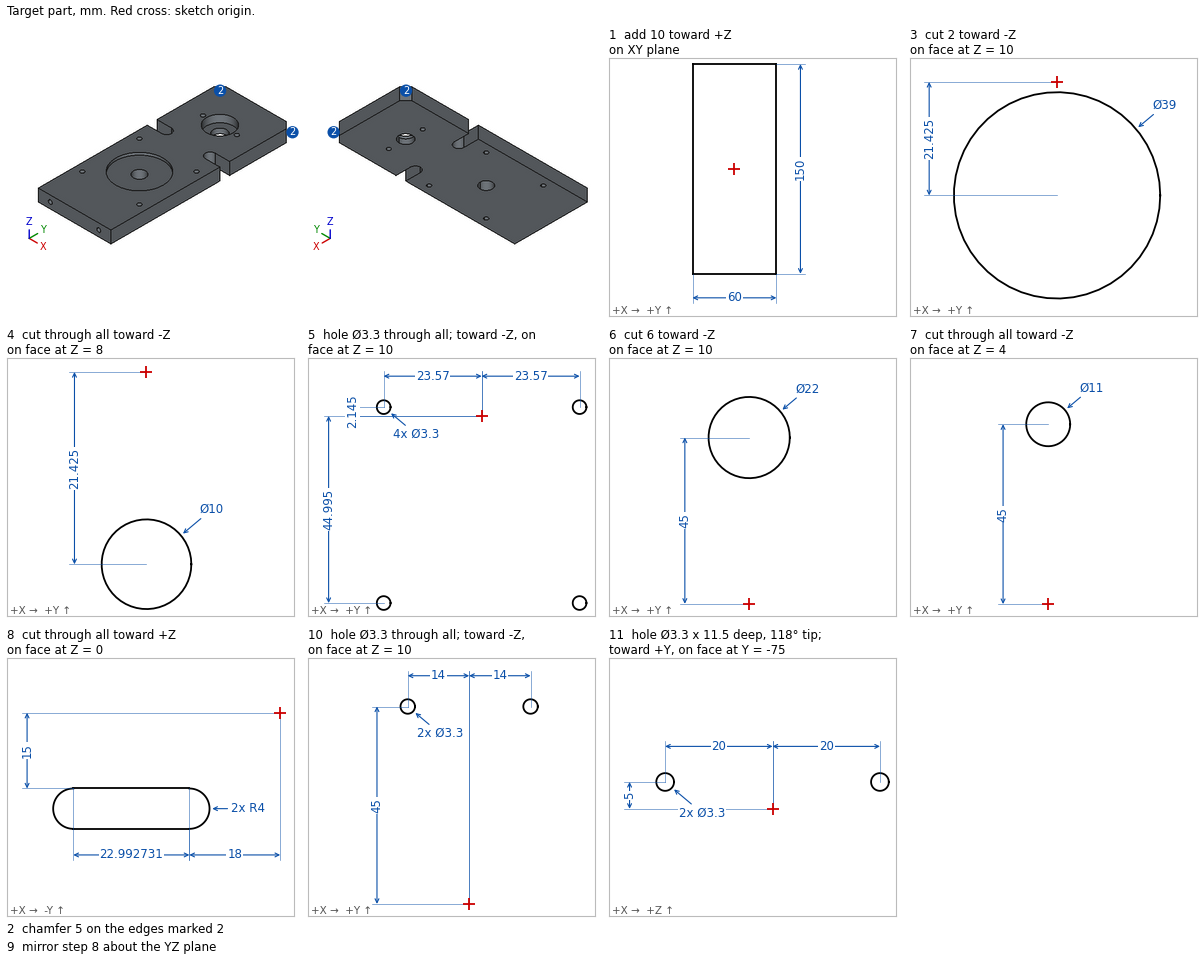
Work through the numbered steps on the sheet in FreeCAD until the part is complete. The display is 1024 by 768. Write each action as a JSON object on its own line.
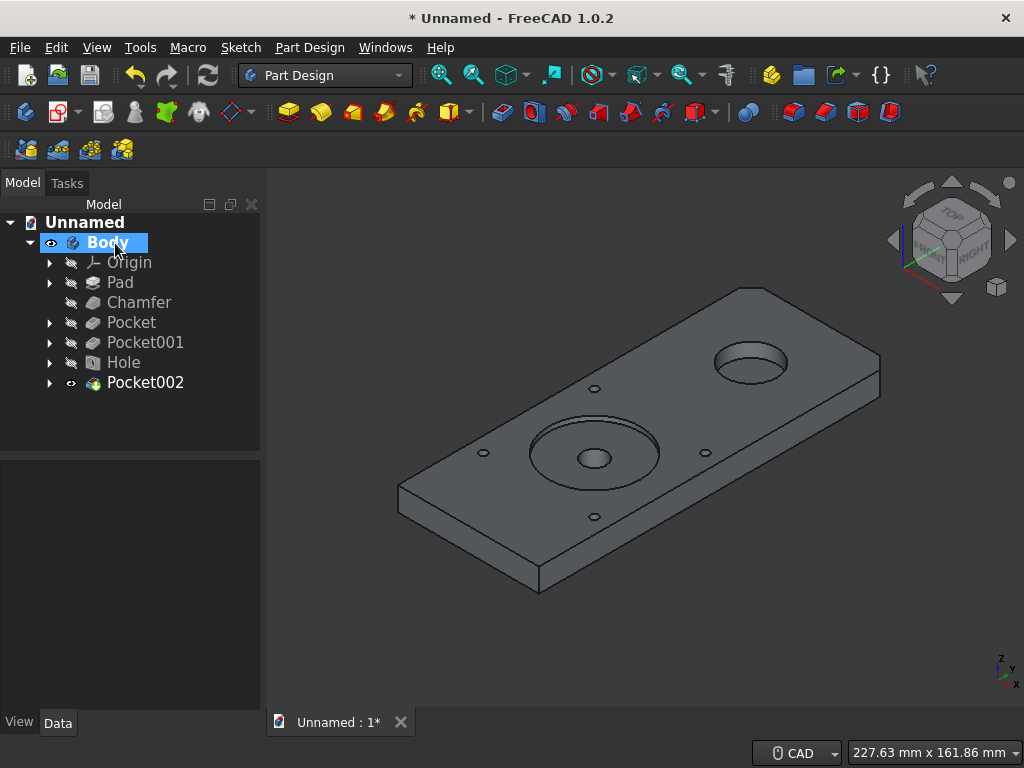
{"action": "left_click", "coordinate": [751, 369]}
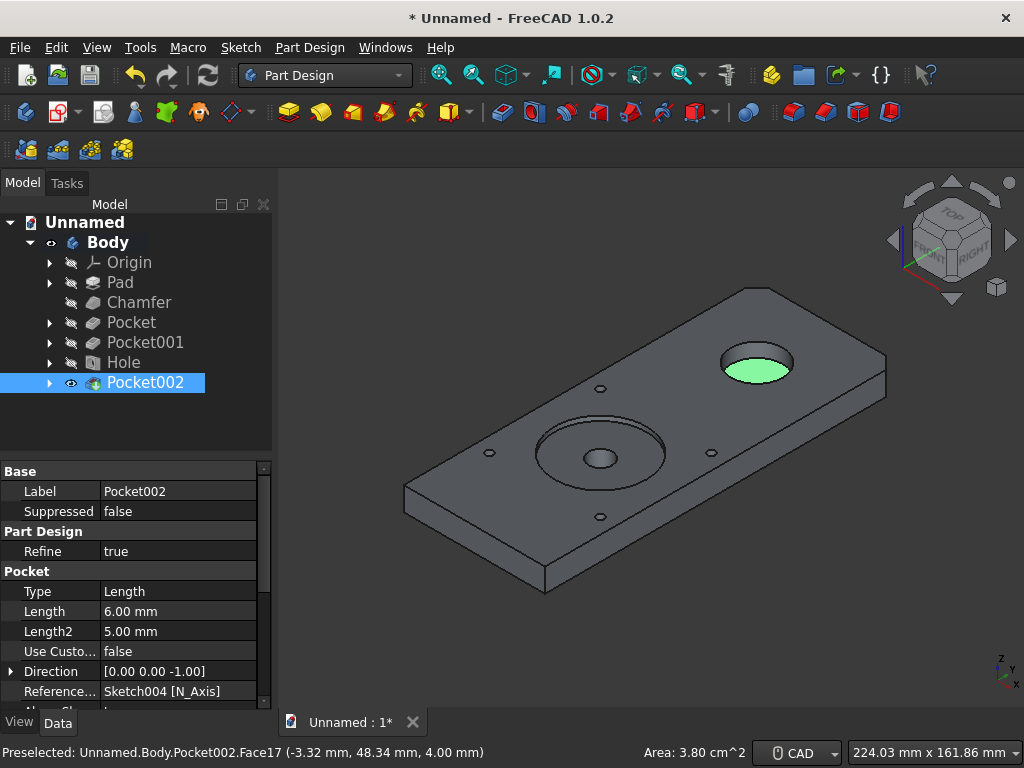
{"action": "left_click", "coordinate": [58, 112]}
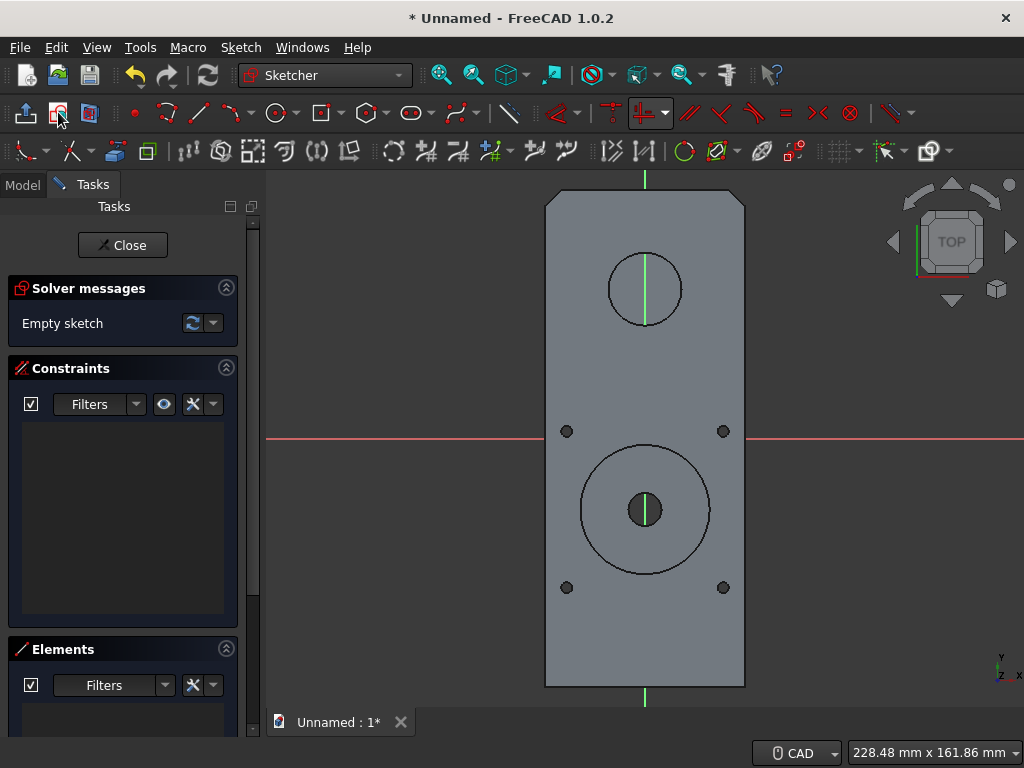
{"action": "left_click", "coordinate": [90, 114]}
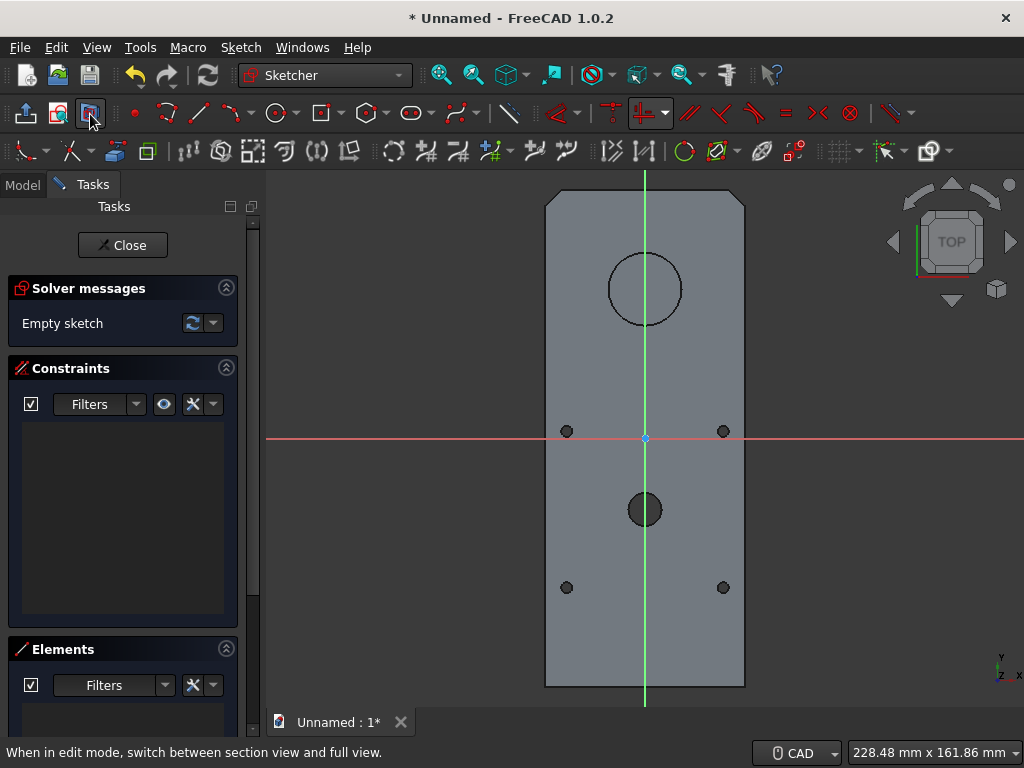
{"action": "scroll", "coordinate": [654, 271], "scroll_direction": "up", "scroll_amount": 11}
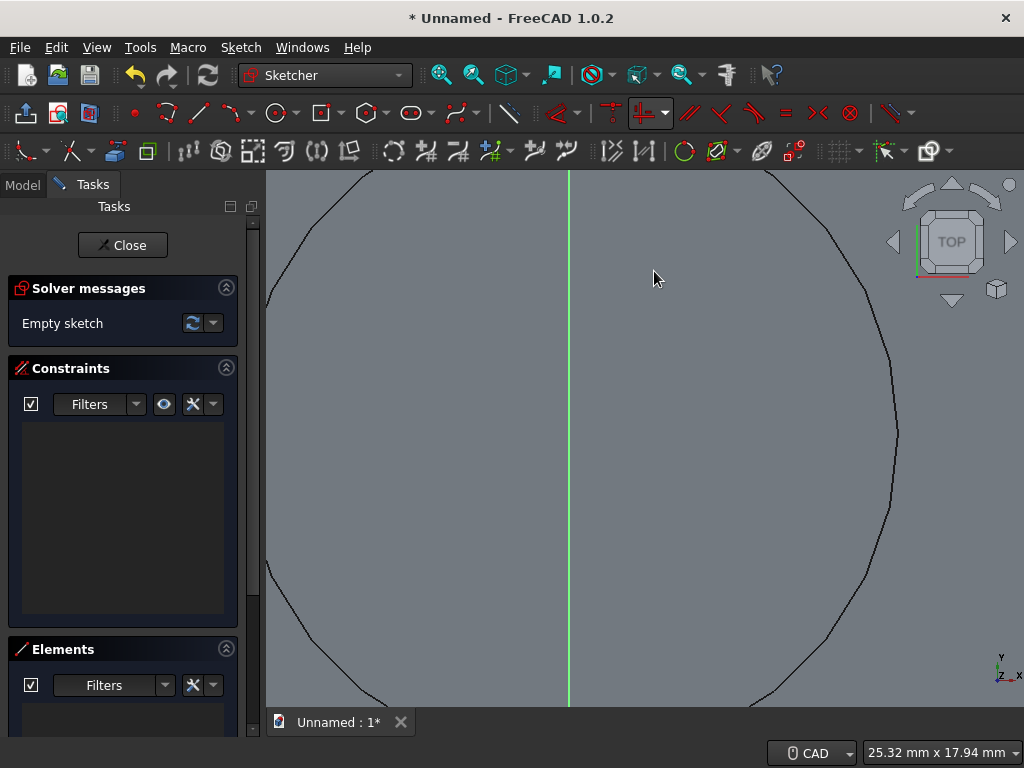
{"action": "key", "text": "g c"}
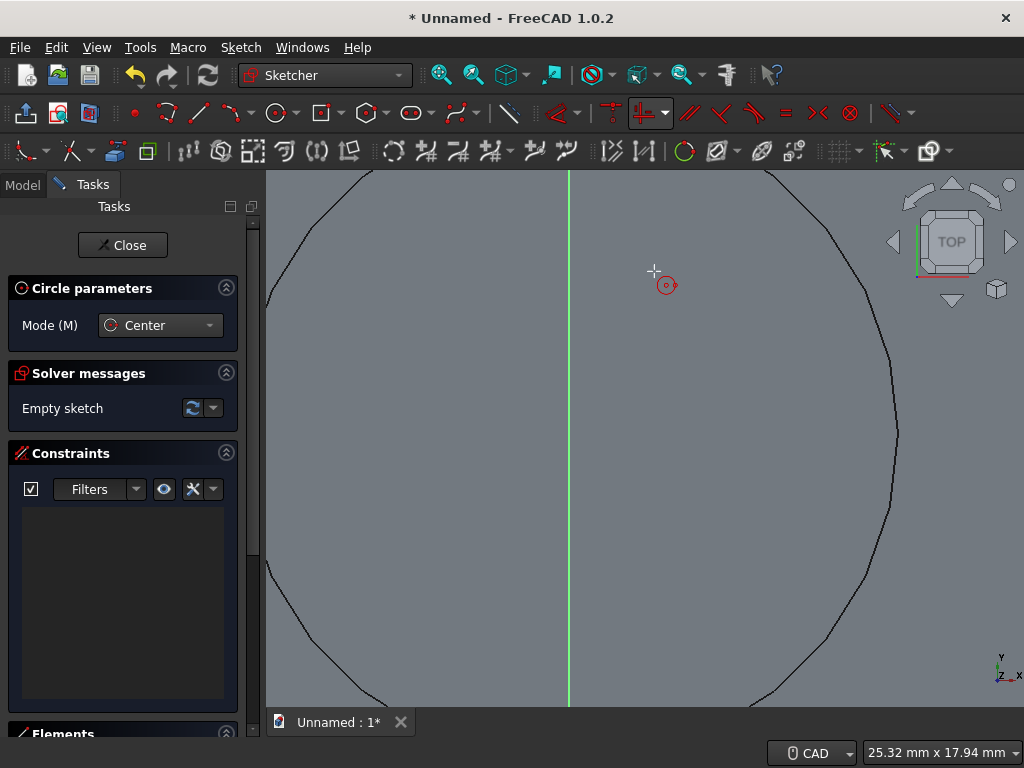
{"action": "left_click", "coordinate": [569, 434]}
{"action": "left_click", "coordinate": [685, 317]}
{"action": "key", "text": "Escape"}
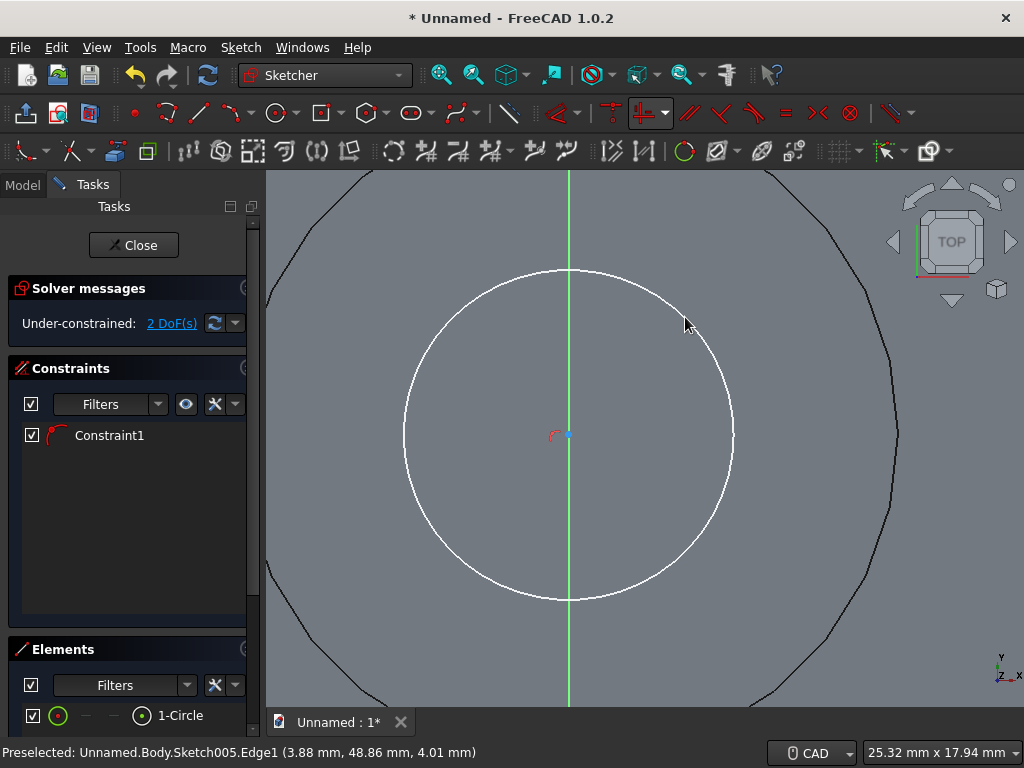
{"action": "key", "text": "d"}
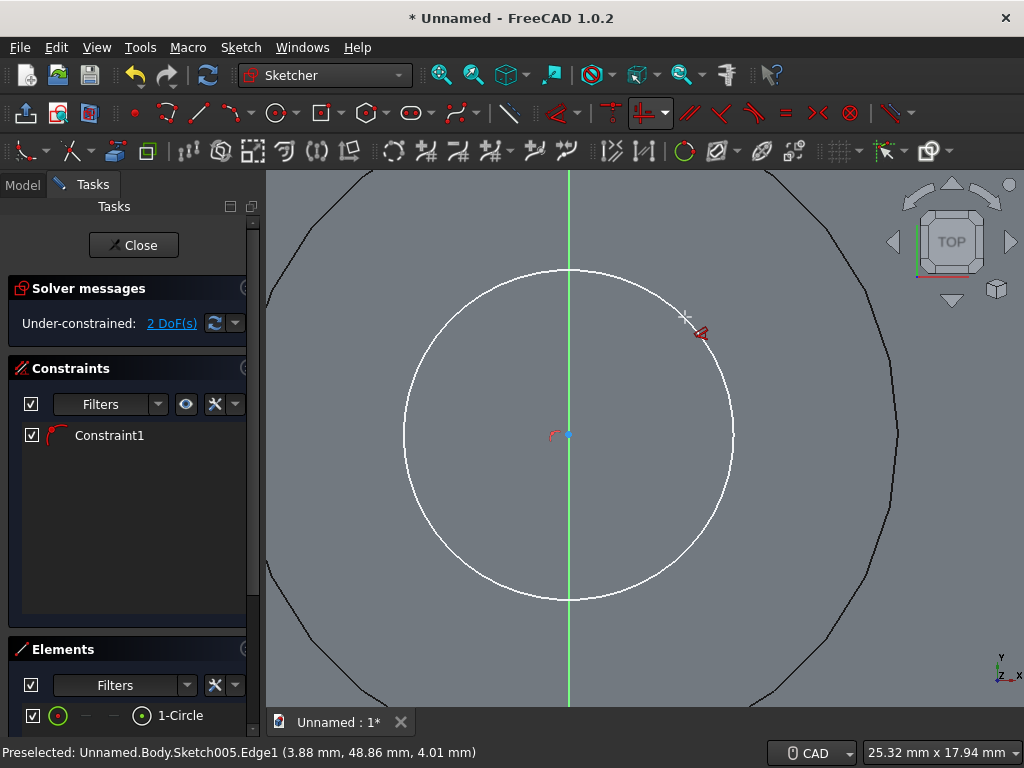
{"action": "left_click", "coordinate": [685, 318]}
{"action": "left_click", "coordinate": [708, 295]}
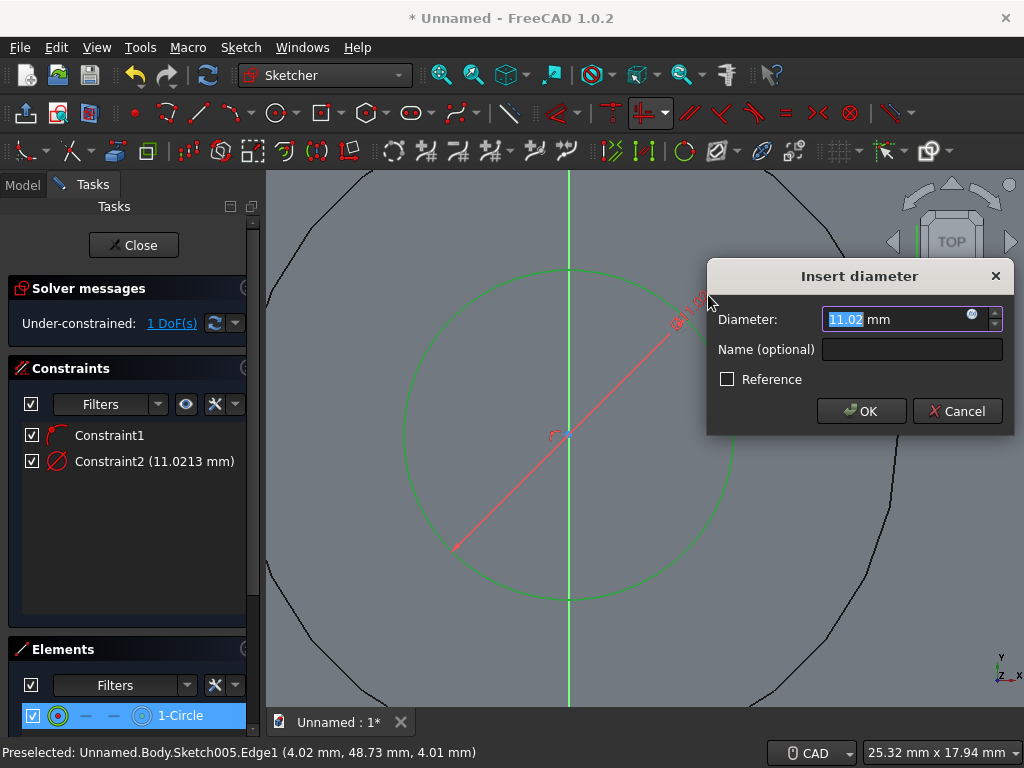
{"action": "type", "text": "11"}
{"action": "key", "text": "Return"}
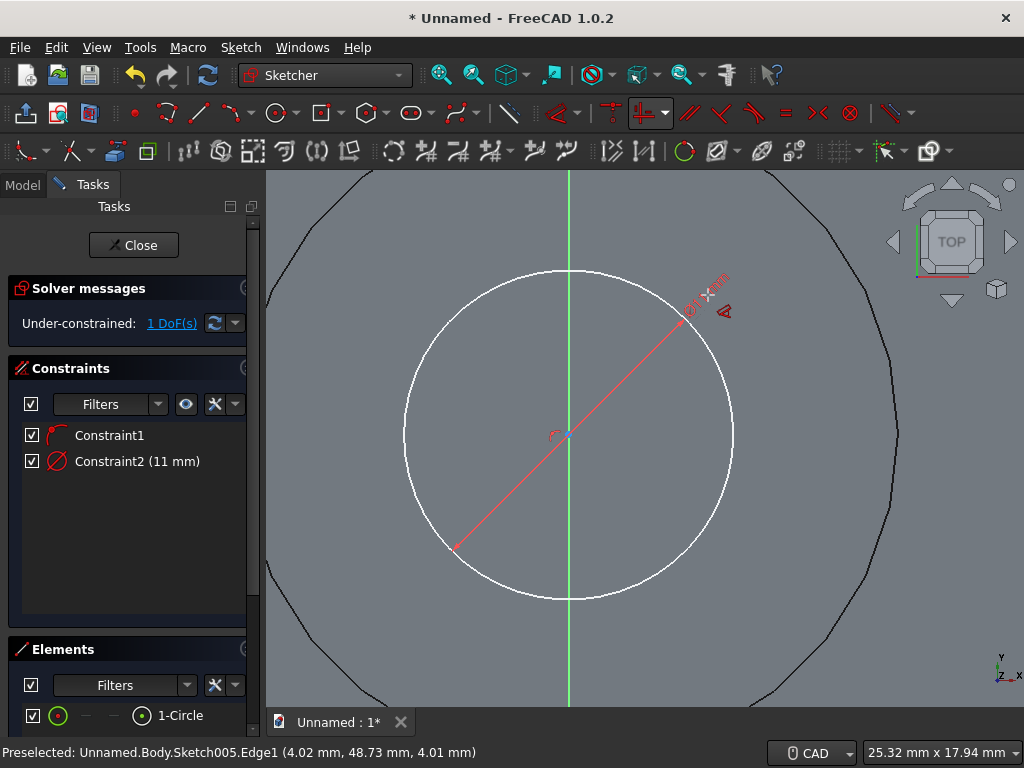
{"action": "left_click", "coordinate": [569, 435]}
{"action": "left_click", "coordinate": [603, 557]}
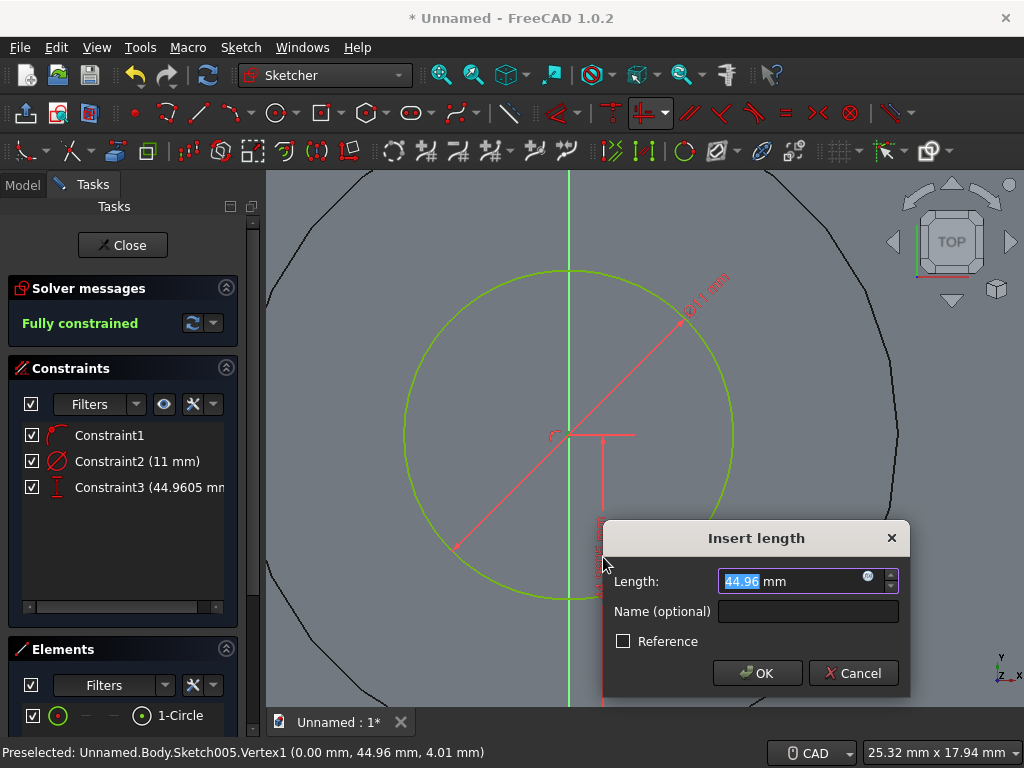
{"action": "type", "text": "45"}
{"action": "key", "text": "Return"}
{"action": "key", "text": "Escape"}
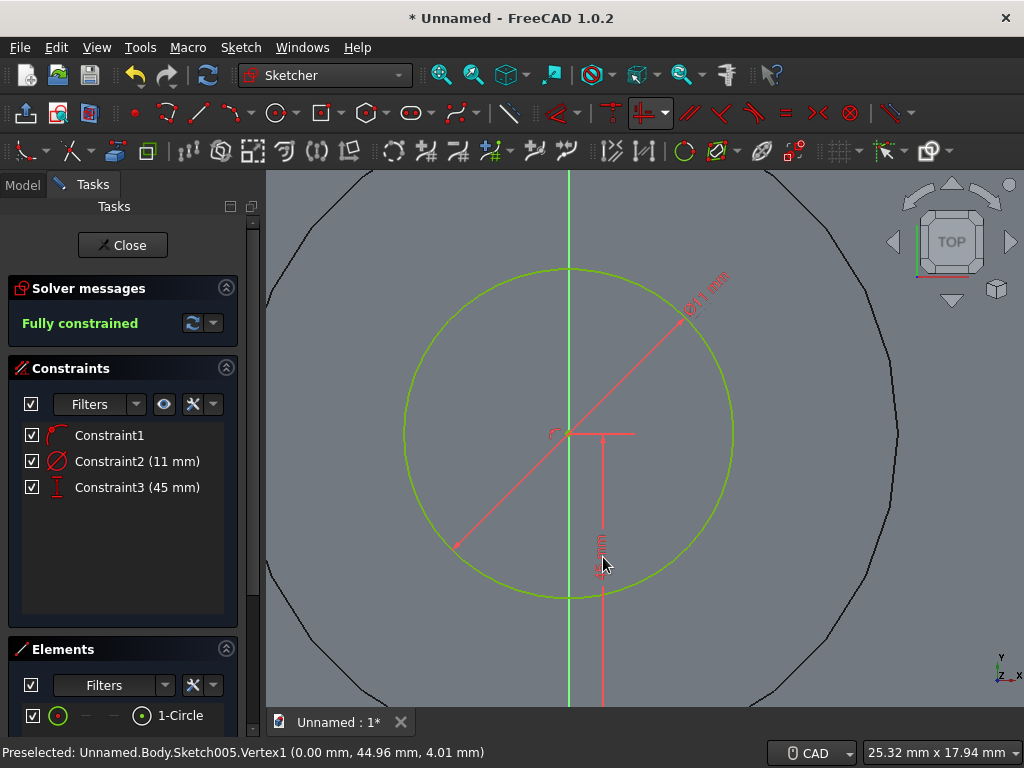
{"action": "left_click", "coordinate": [123, 245]}